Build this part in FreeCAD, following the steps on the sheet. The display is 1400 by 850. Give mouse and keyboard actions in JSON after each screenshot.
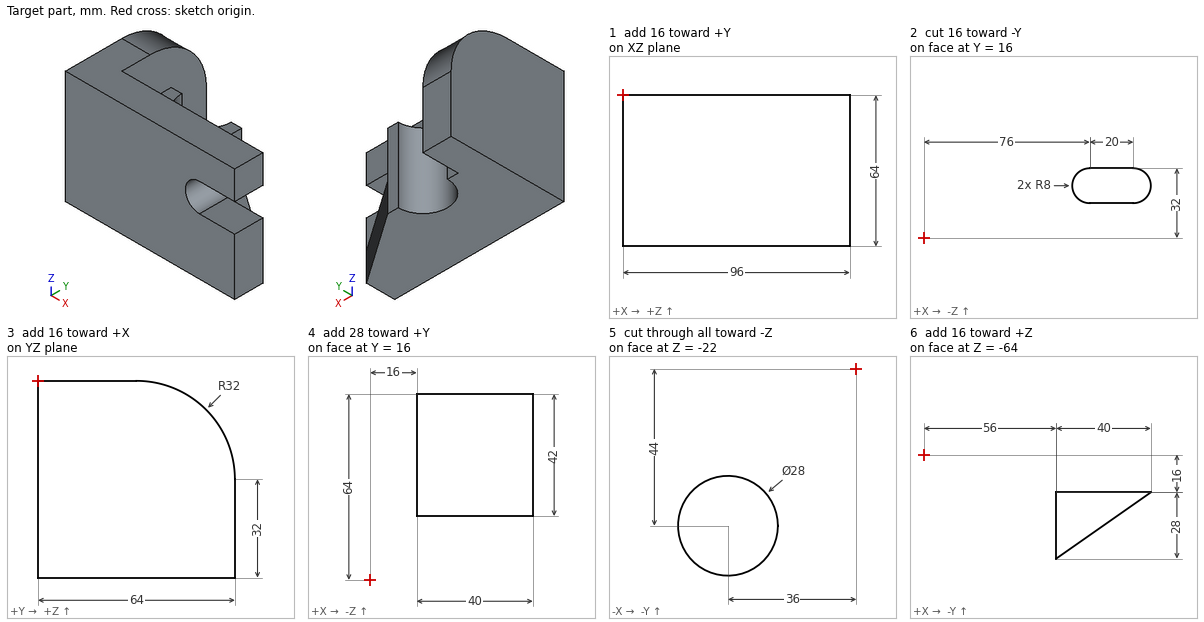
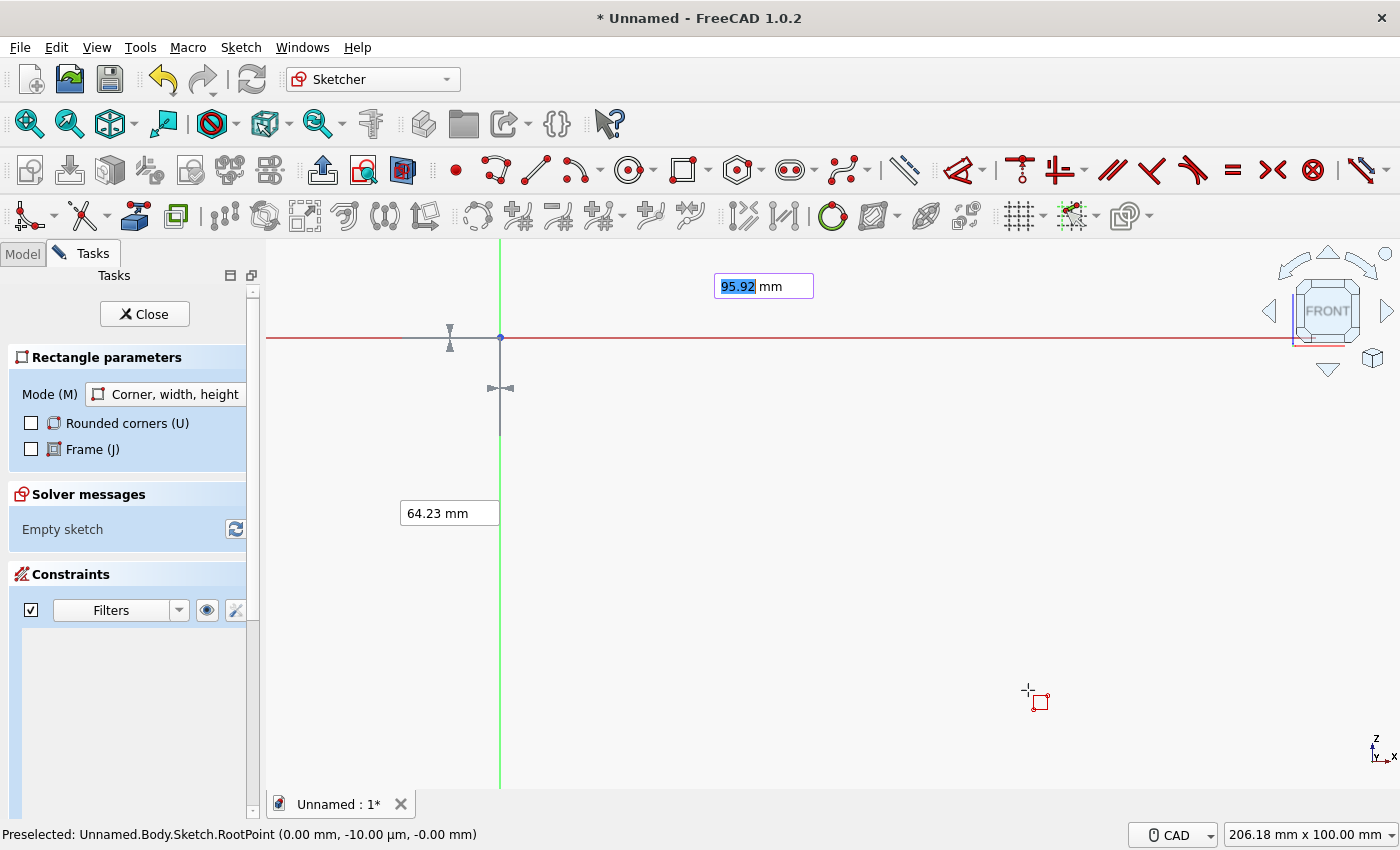
{"action": "type", "text": "96"}
{"action": "key", "text": "Tab"}
{"action": "type", "text": "64"}
{"action": "key", "text": "Return"}
{"action": "key", "text": "Escape"}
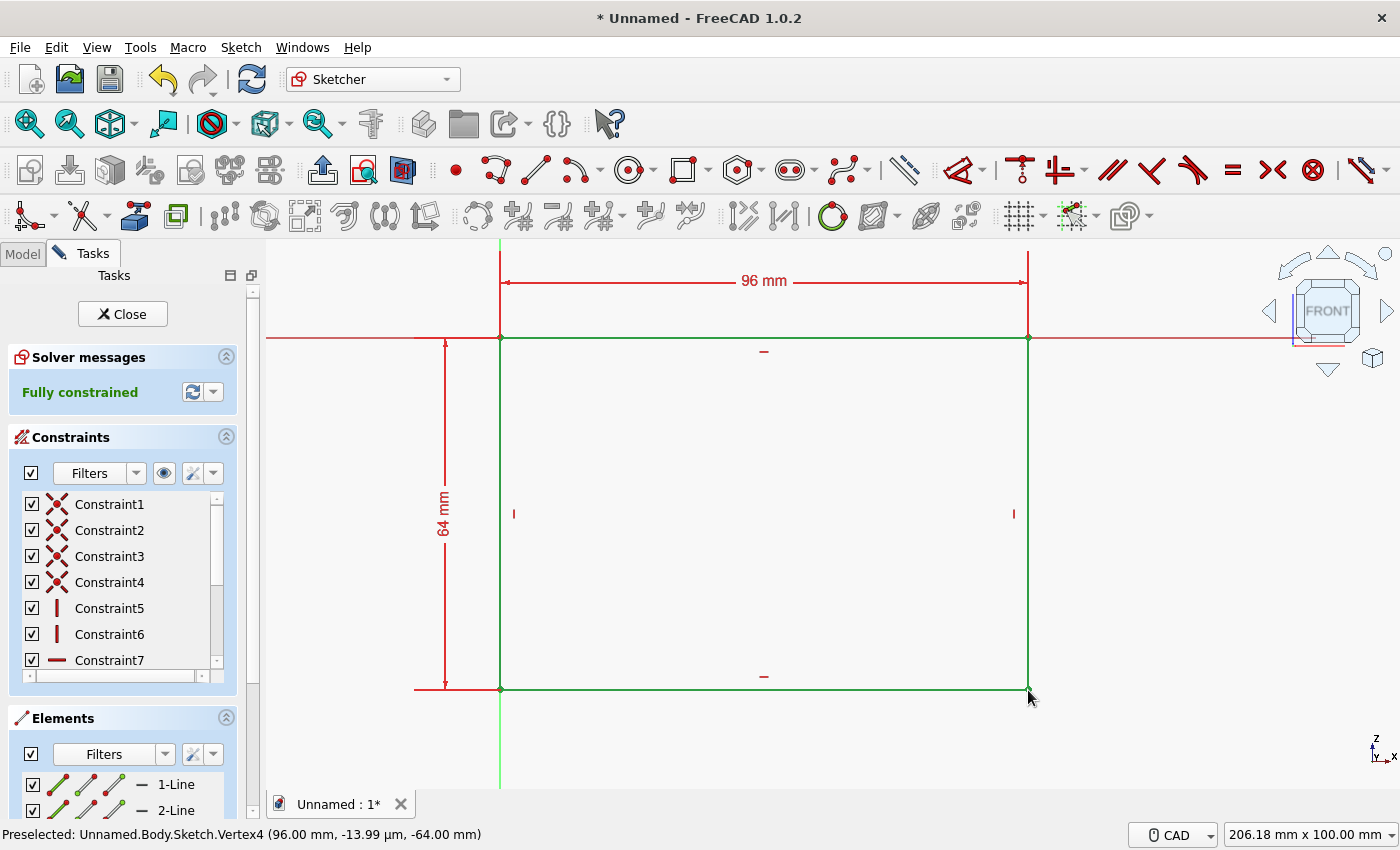
{"action": "left_click", "coordinate": [123, 314]}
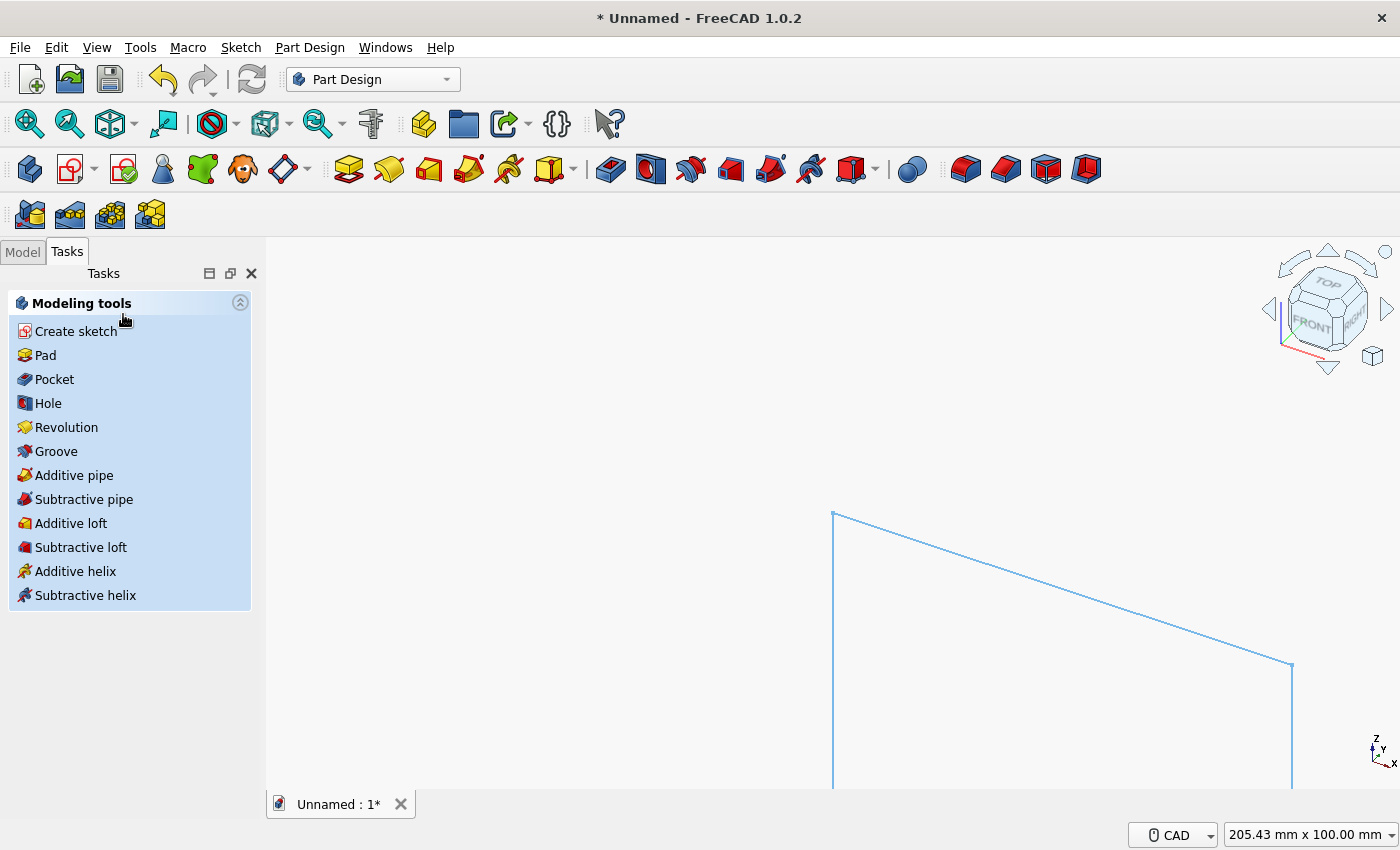
{"action": "left_click", "coordinate": [350, 170]}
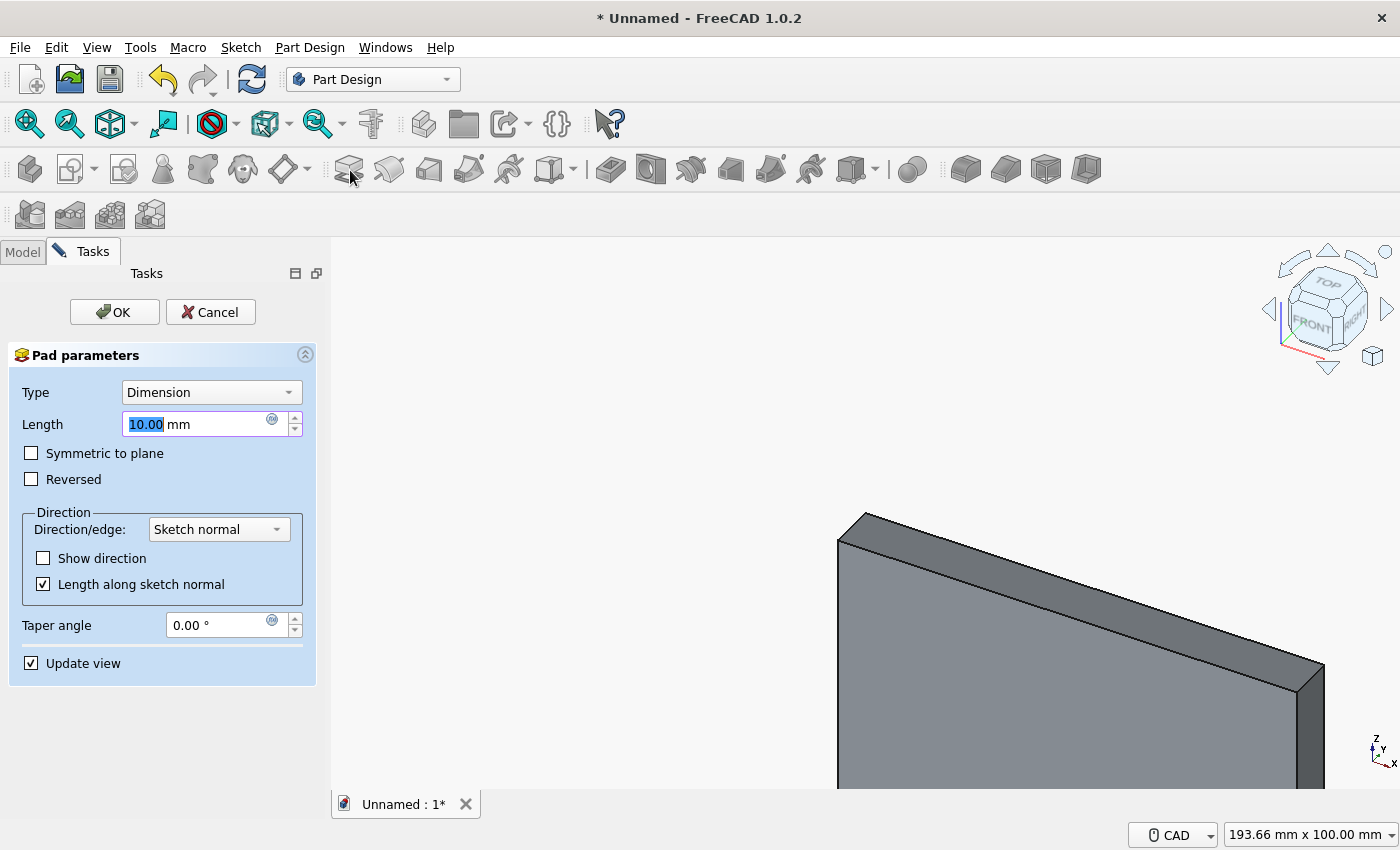
{"action": "type", "text": "16"}
{"action": "key", "text": "Tab"}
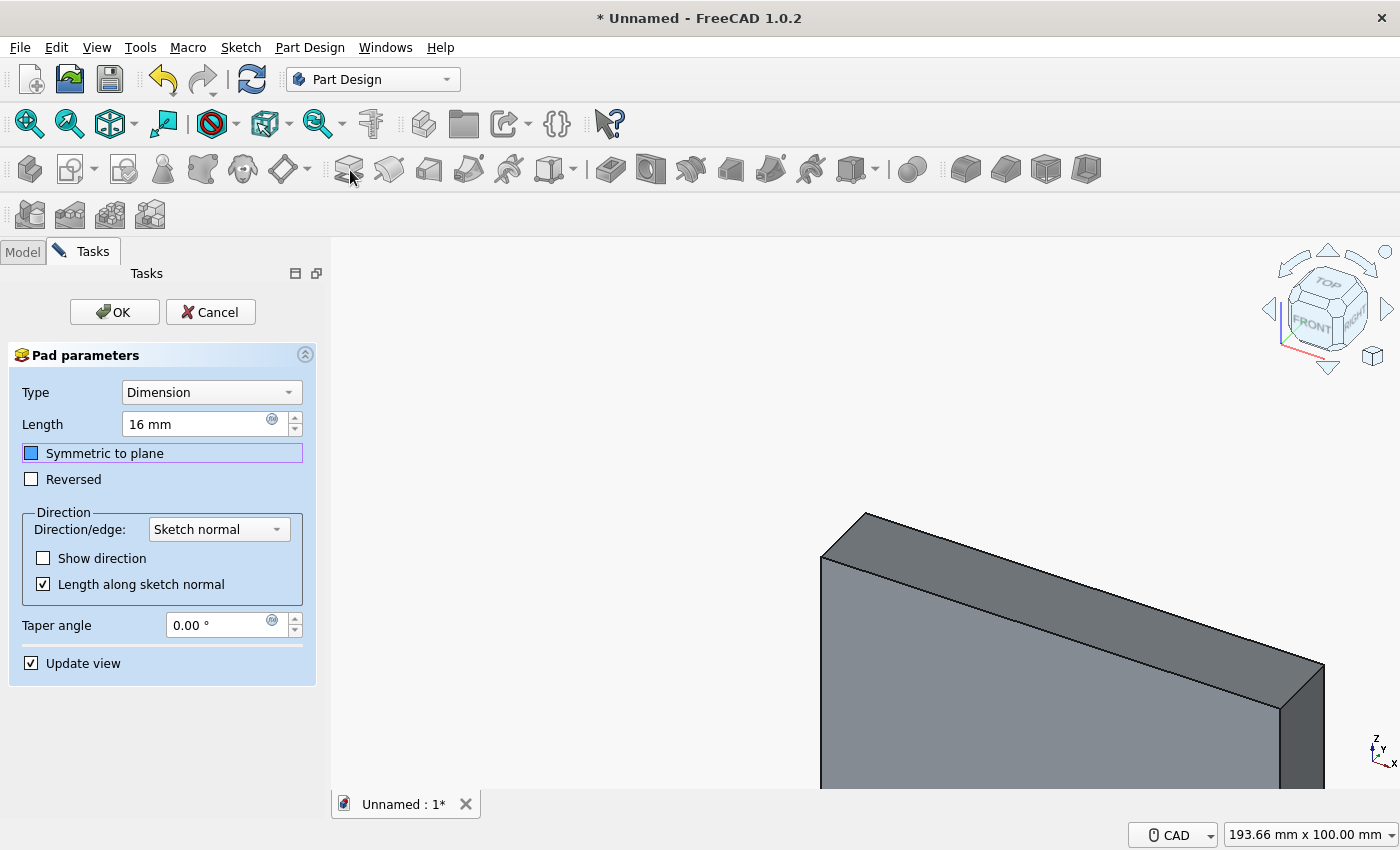
{"action": "left_click", "coordinate": [30, 479]}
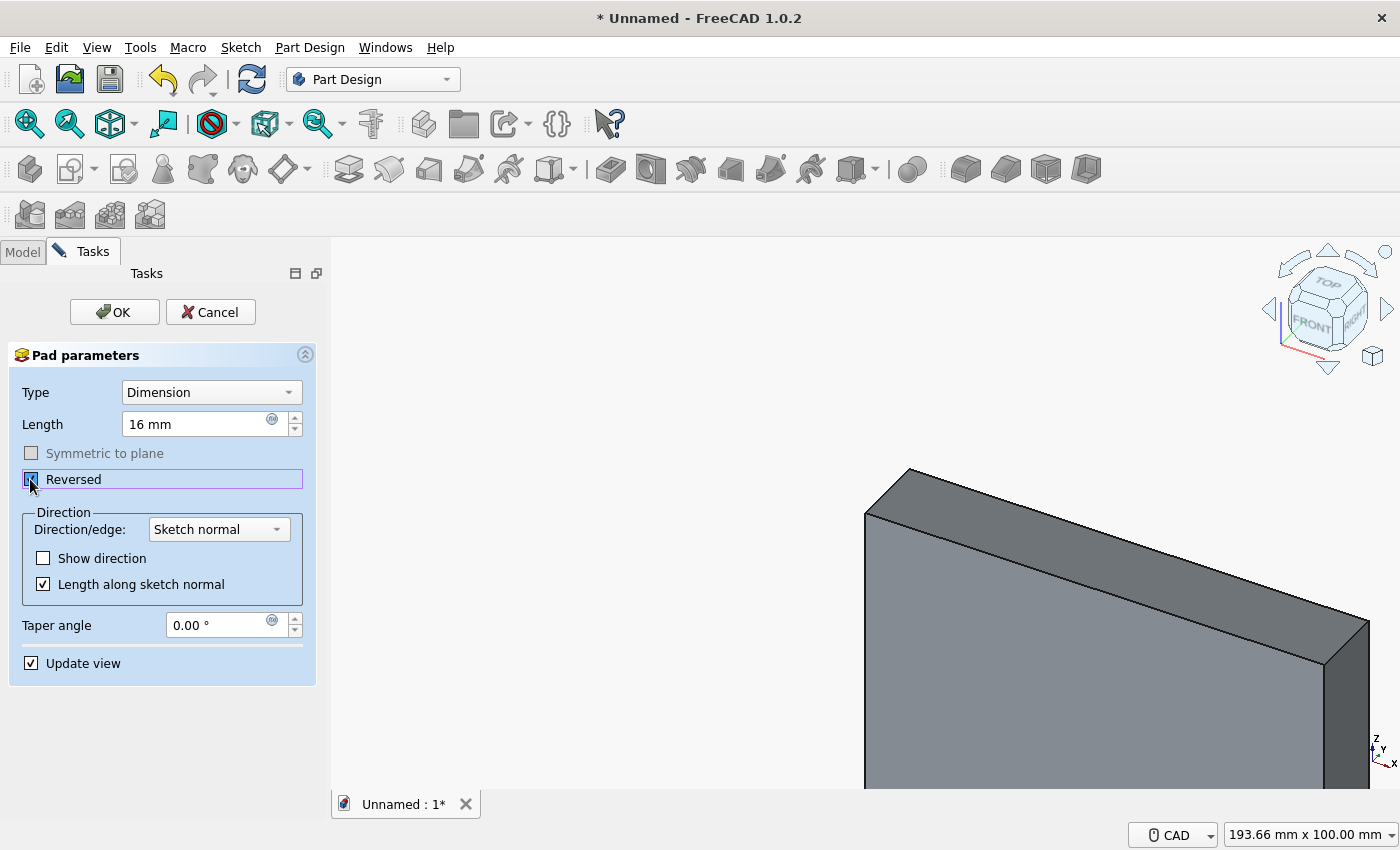
{"action": "left_click", "coordinate": [115, 312]}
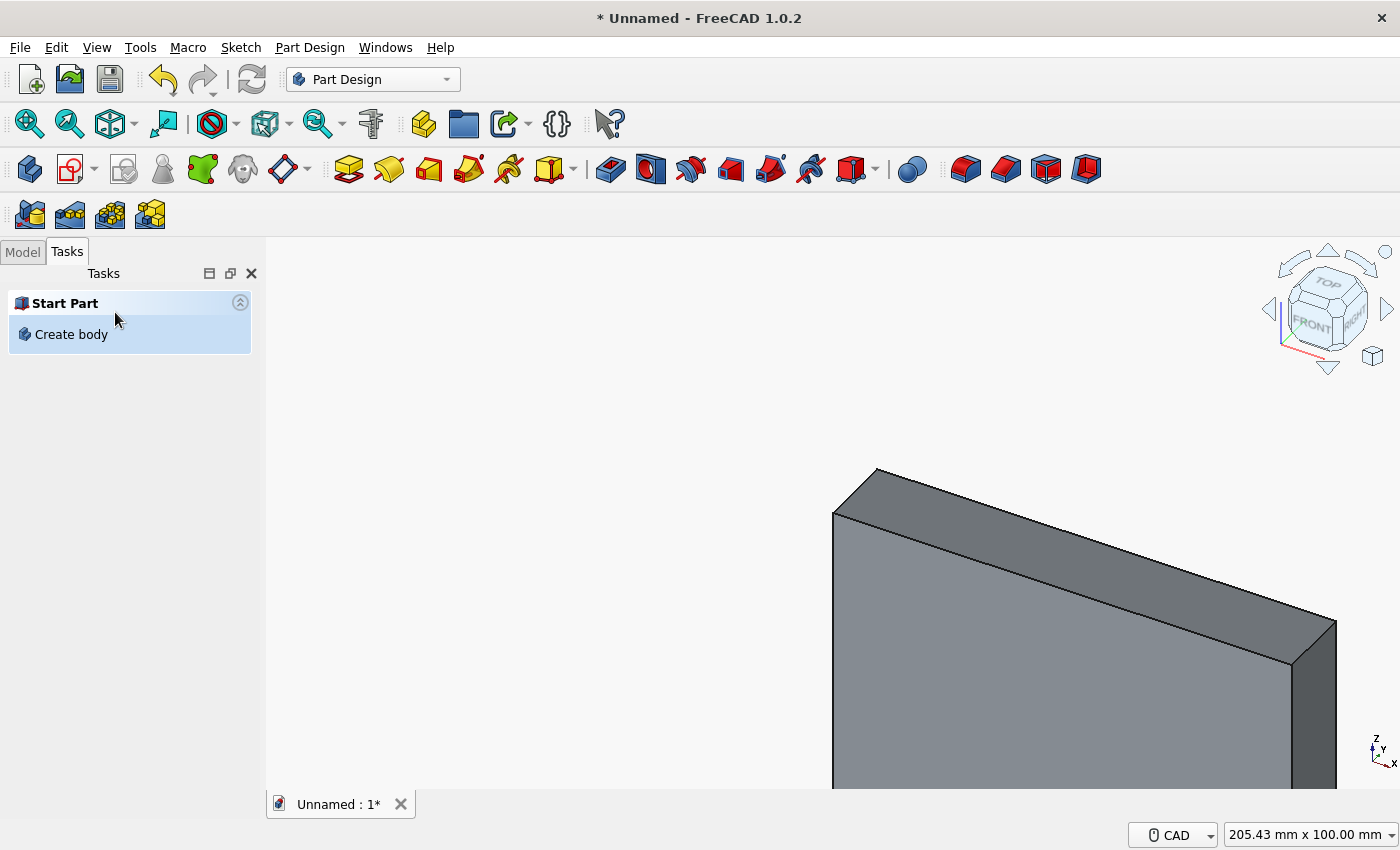
{"action": "left_click", "coordinate": [30, 124]}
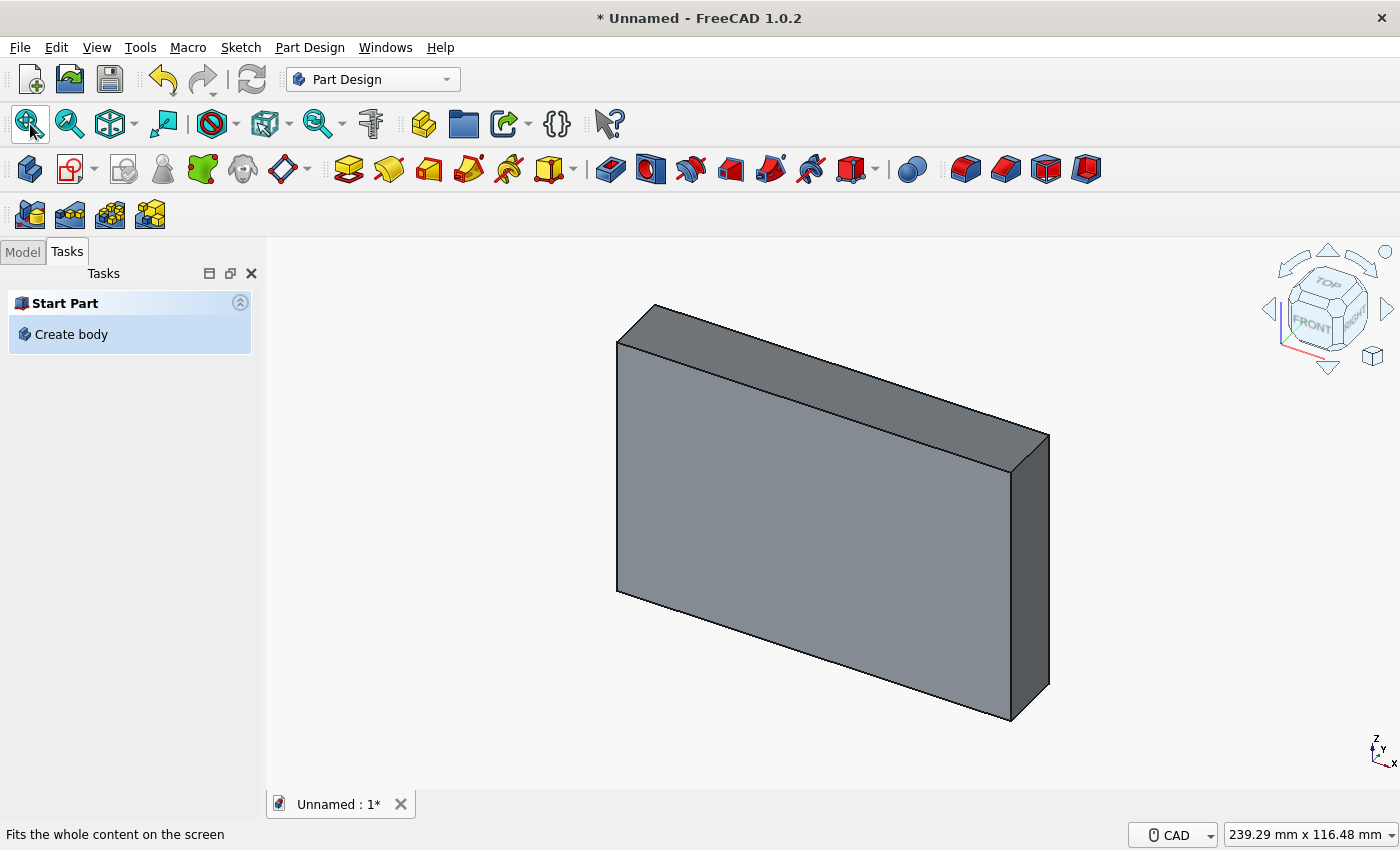
{"action": "key", "text": "4"}